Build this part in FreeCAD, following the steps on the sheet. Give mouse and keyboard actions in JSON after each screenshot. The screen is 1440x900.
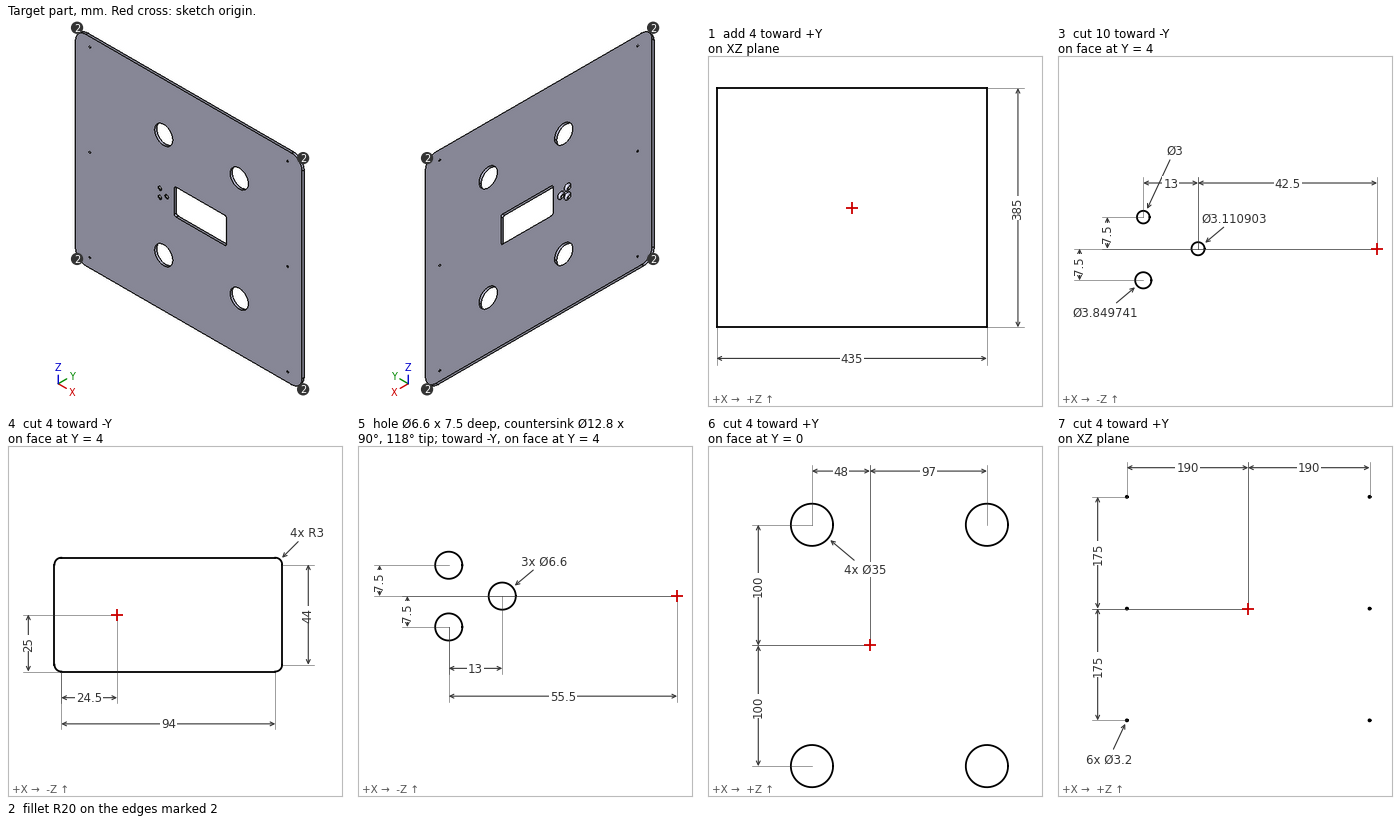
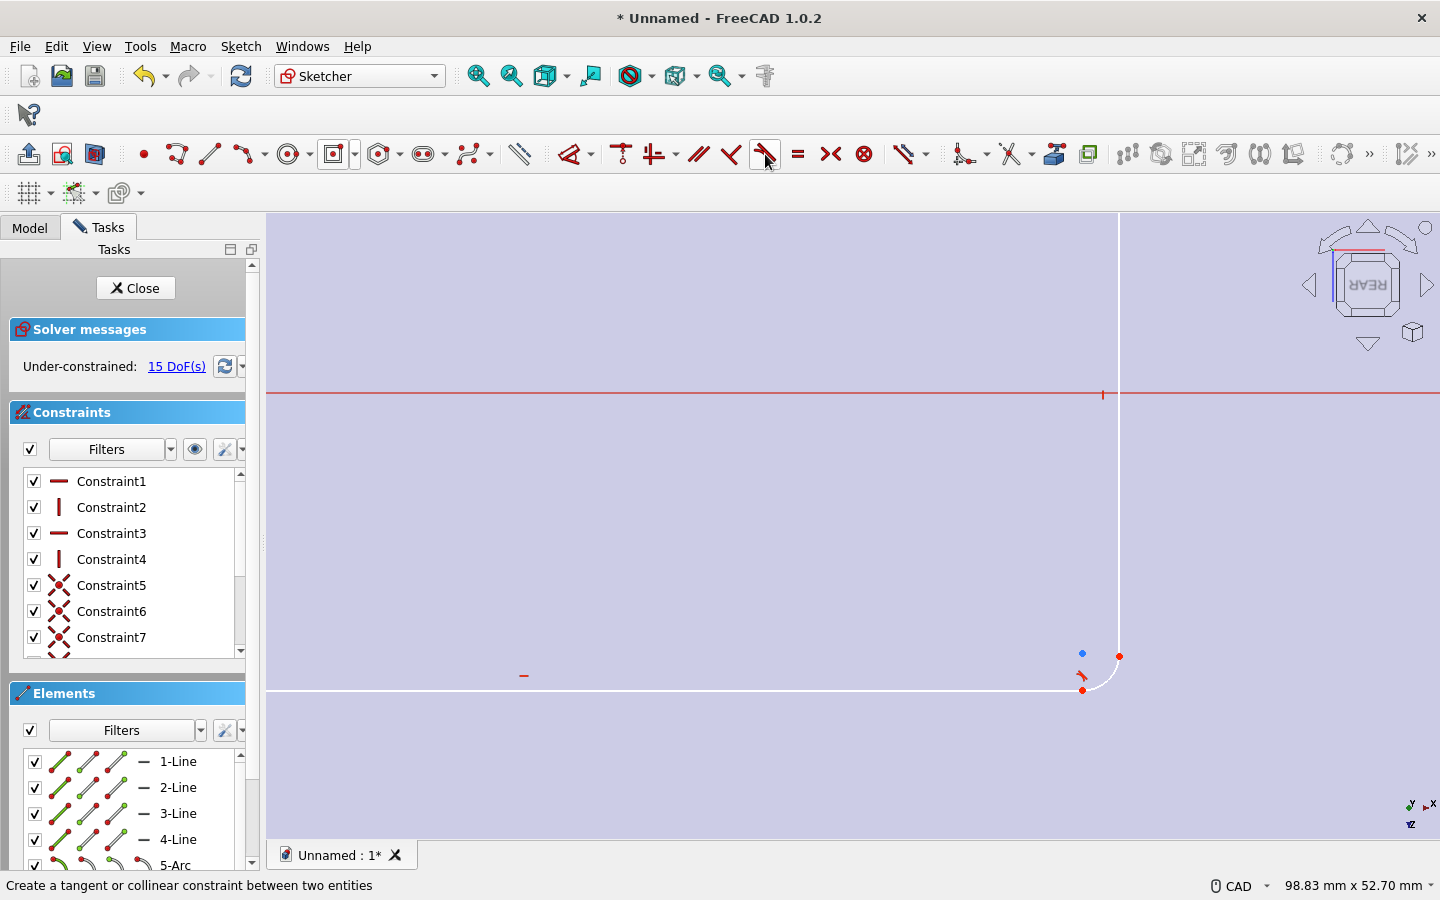
{"action": "left_click", "coordinate": [301, 691]}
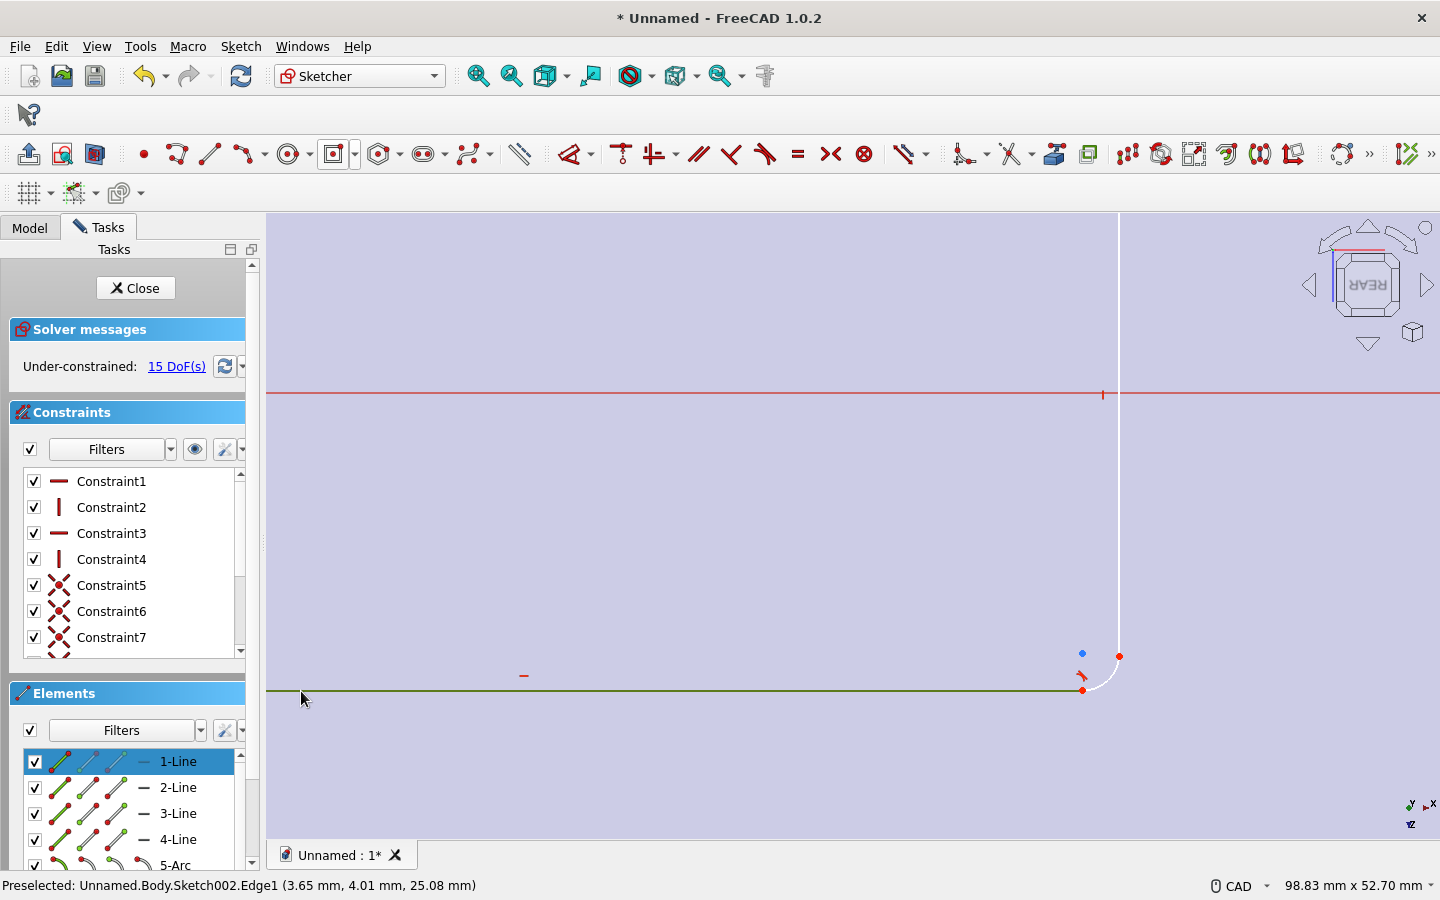
{"action": "scroll", "coordinate": [1100, 688], "scroll_direction": "down", "scroll_amount": 3}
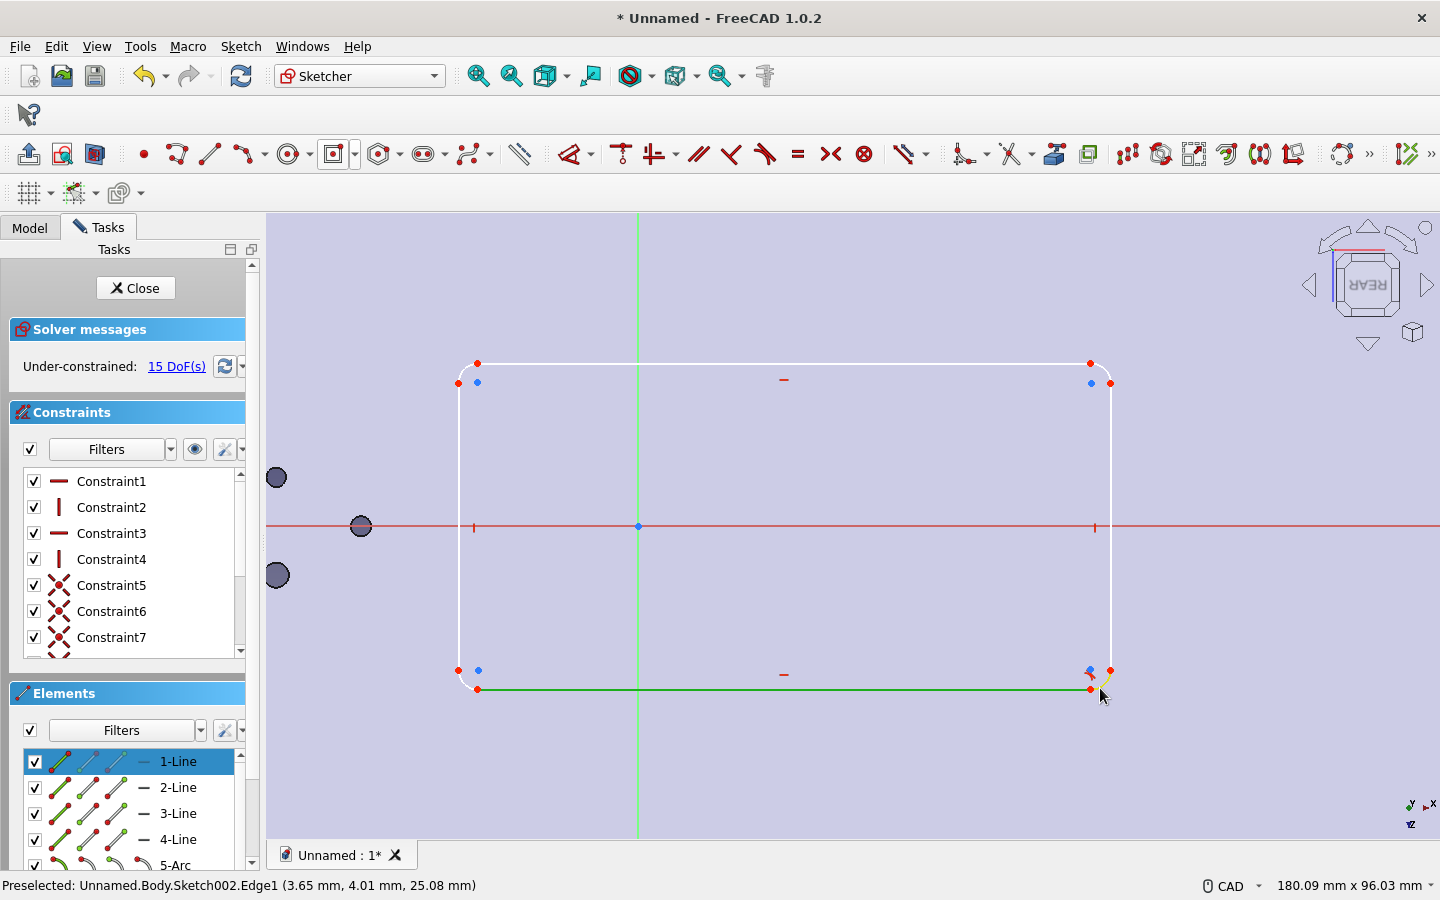
{"action": "scroll", "coordinate": [461, 679], "scroll_direction": "up", "scroll_amount": 3}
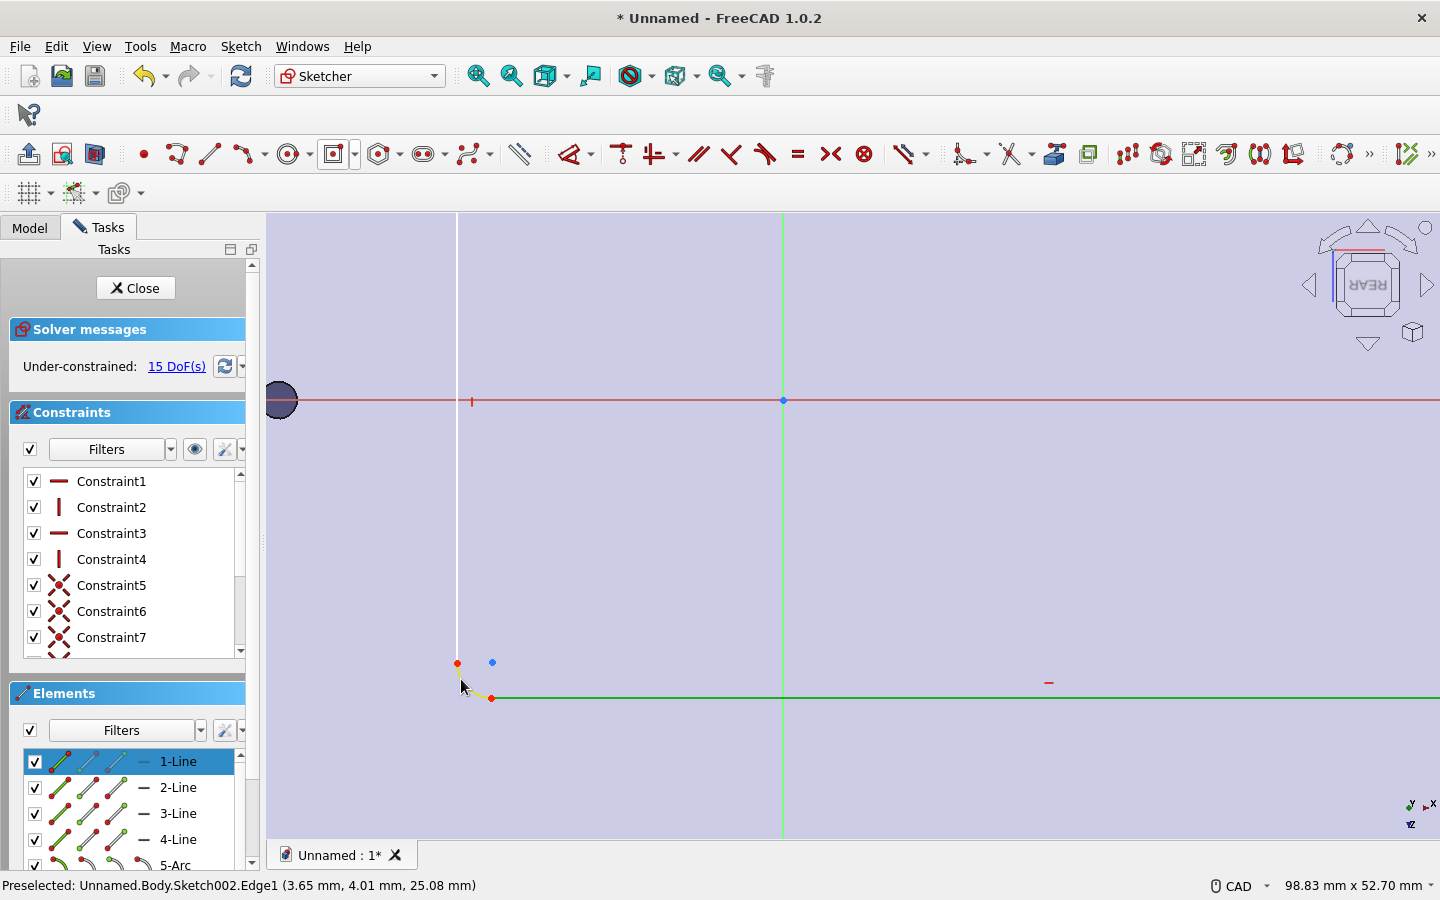
{"action": "left_click", "coordinate": [461, 679]}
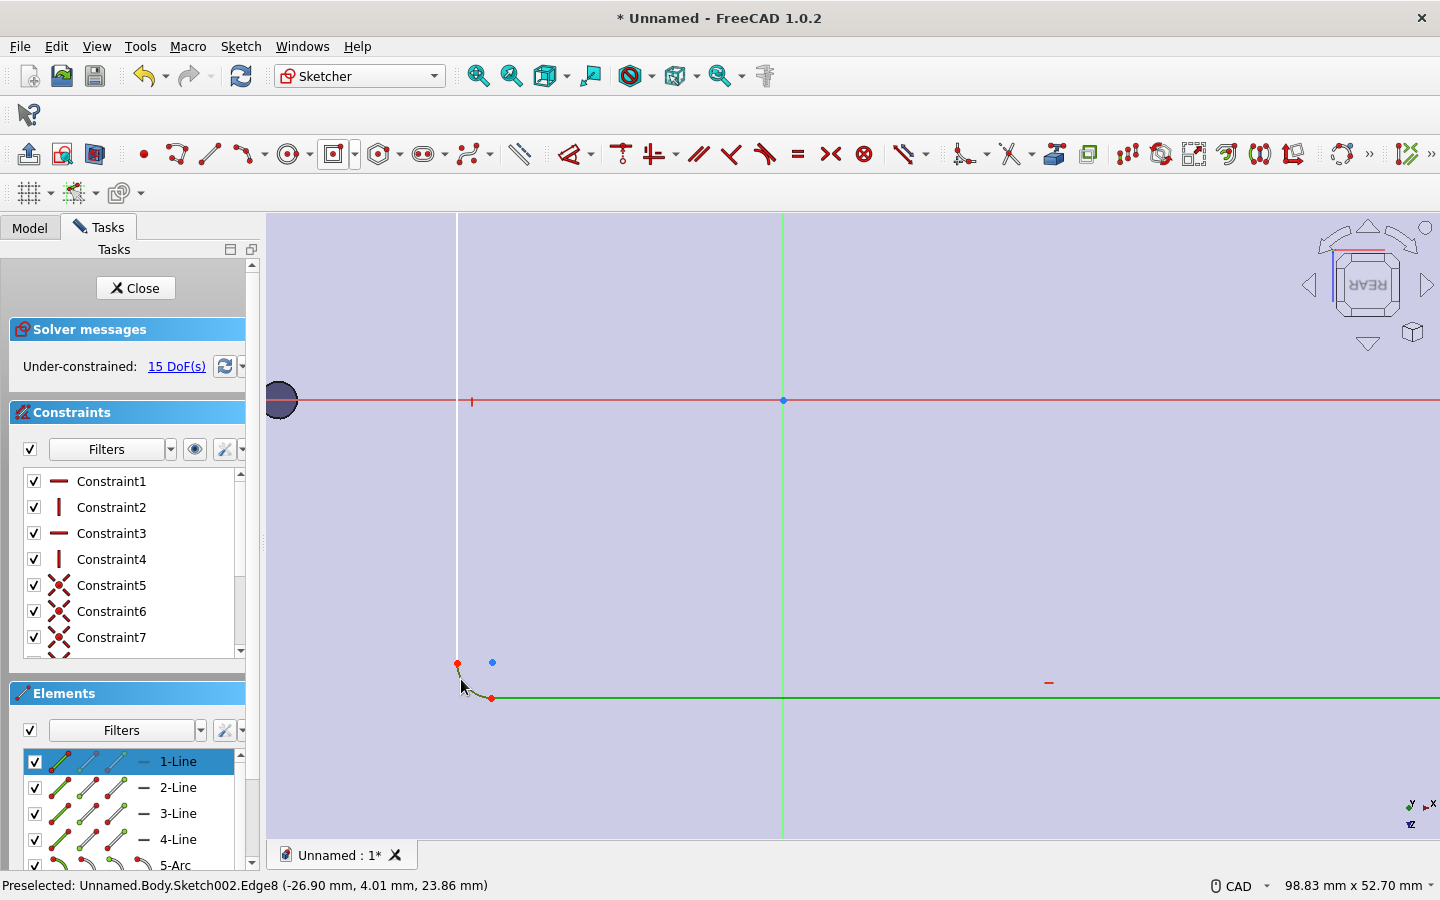
{"action": "left_click", "coordinate": [765, 154]}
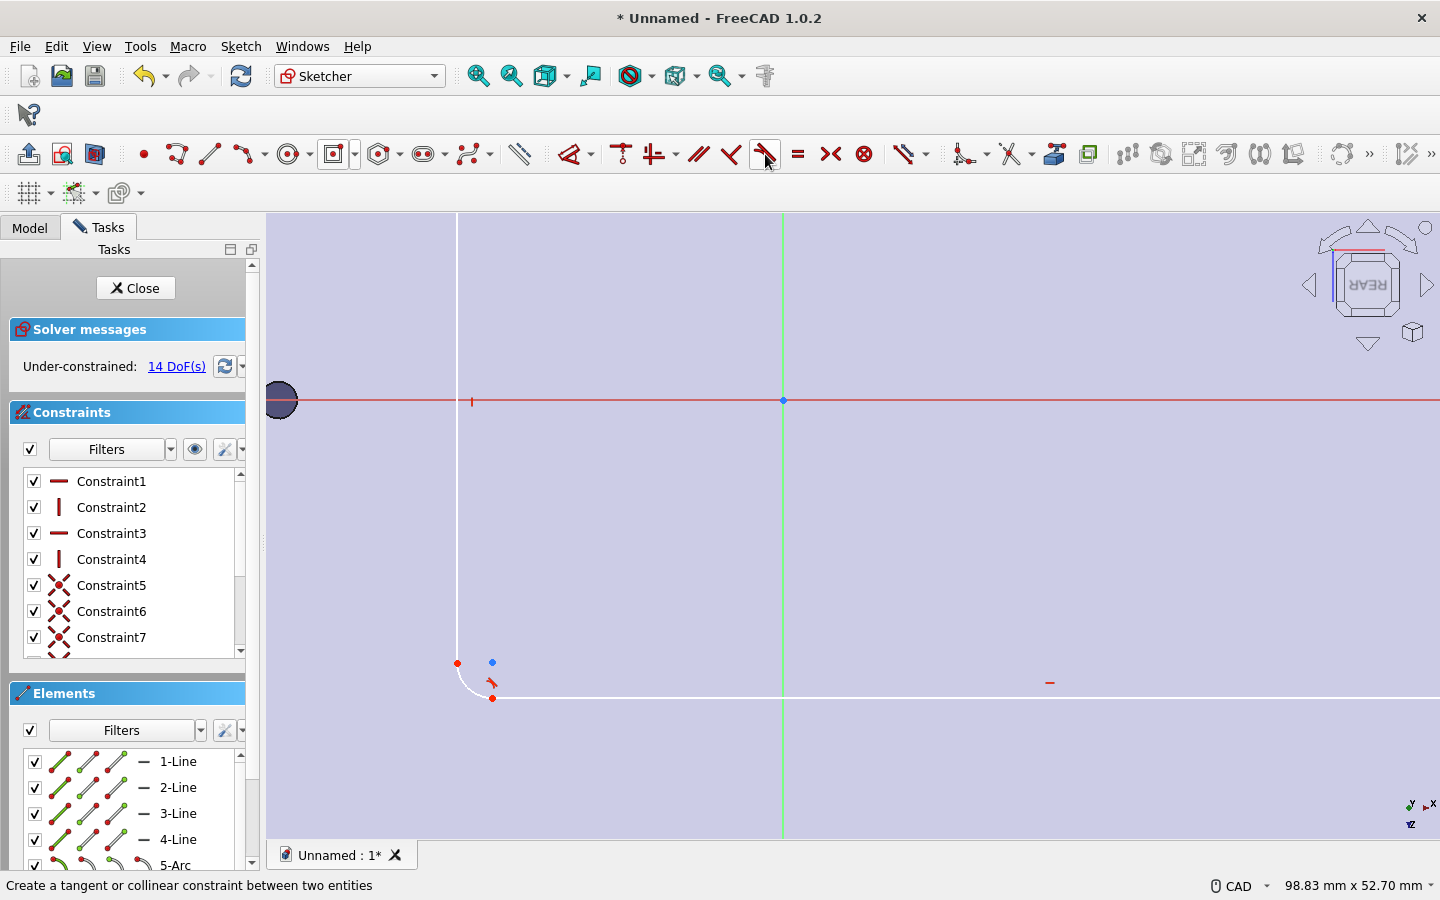
{"action": "scroll", "coordinate": [461, 679], "scroll_direction": "down", "scroll_amount": 3}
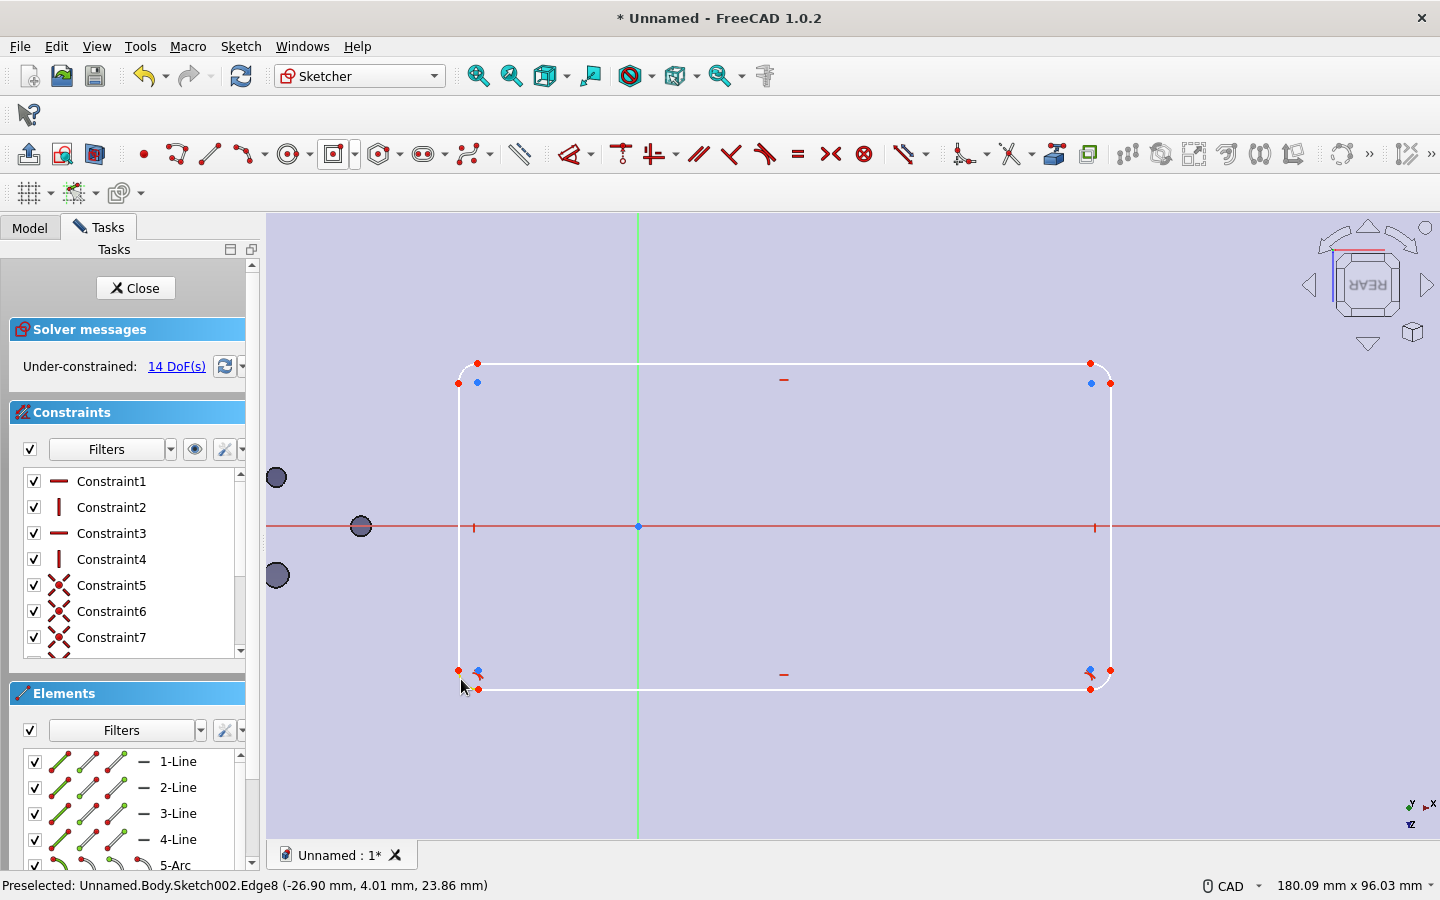
{"action": "left_click", "coordinate": [1111, 585]}